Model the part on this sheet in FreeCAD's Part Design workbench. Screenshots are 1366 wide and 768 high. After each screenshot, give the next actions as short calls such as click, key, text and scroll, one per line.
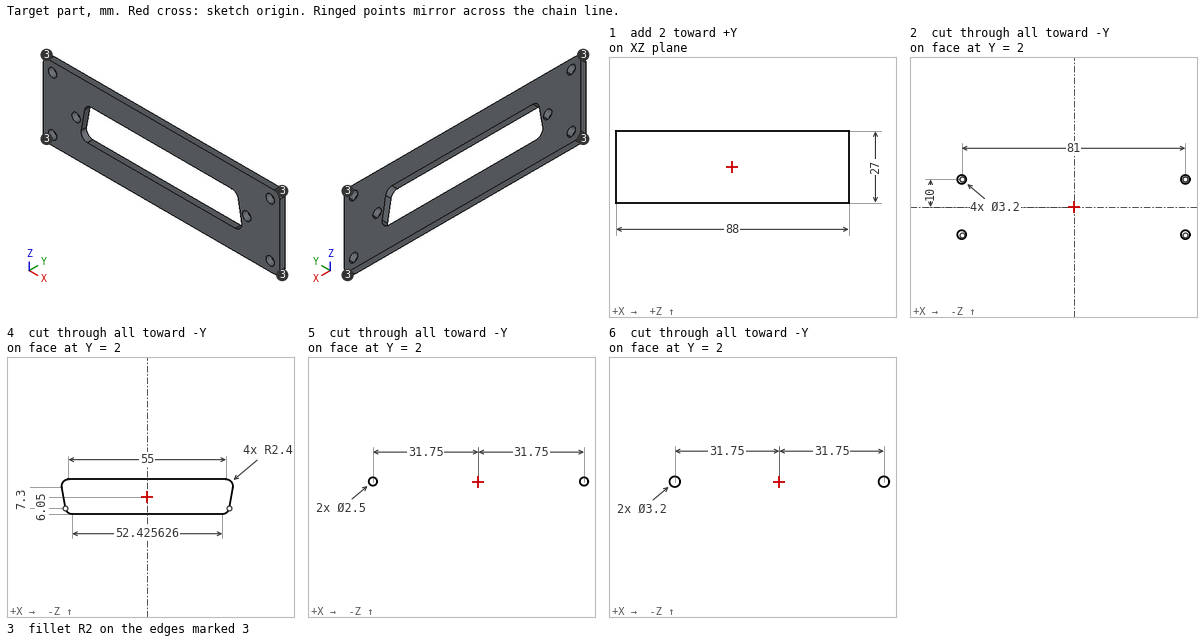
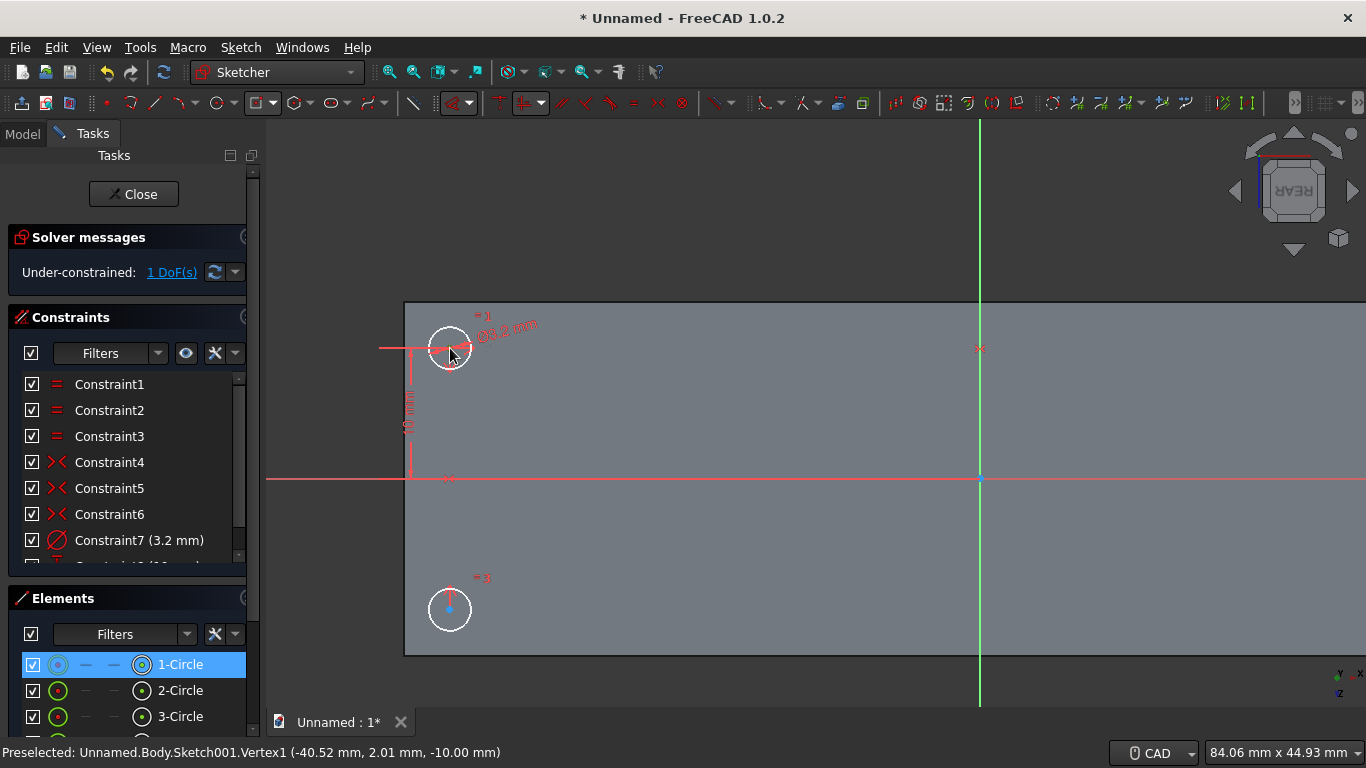
scroll(464, 333, down, 3)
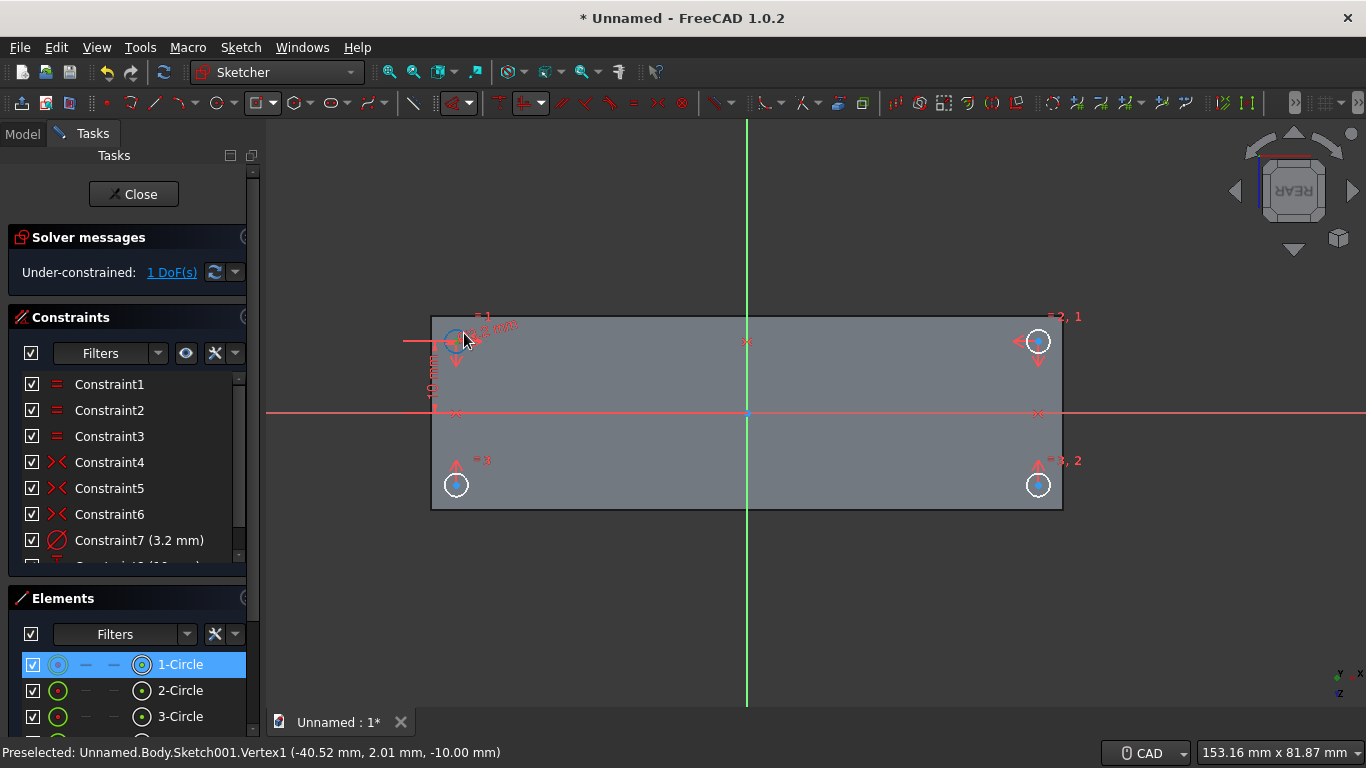
click(1038, 341)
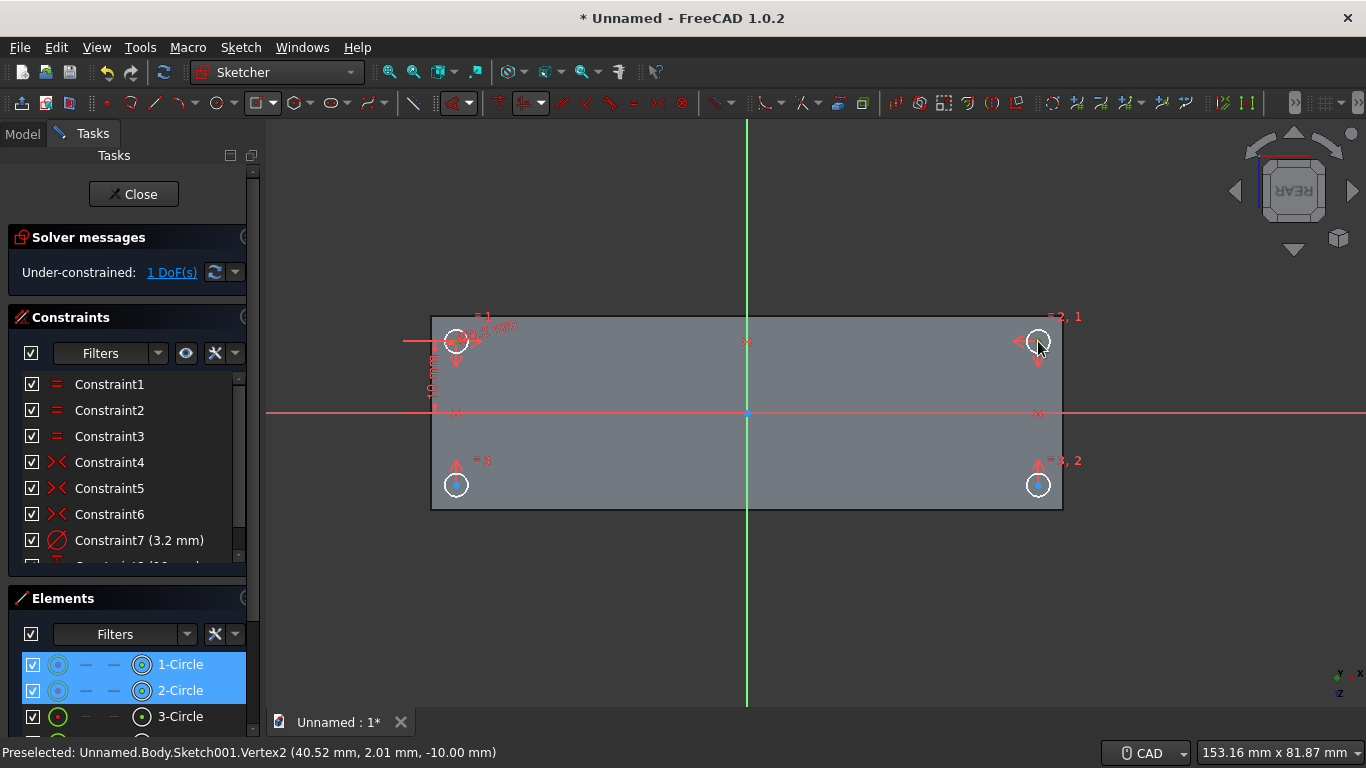
click(472, 104)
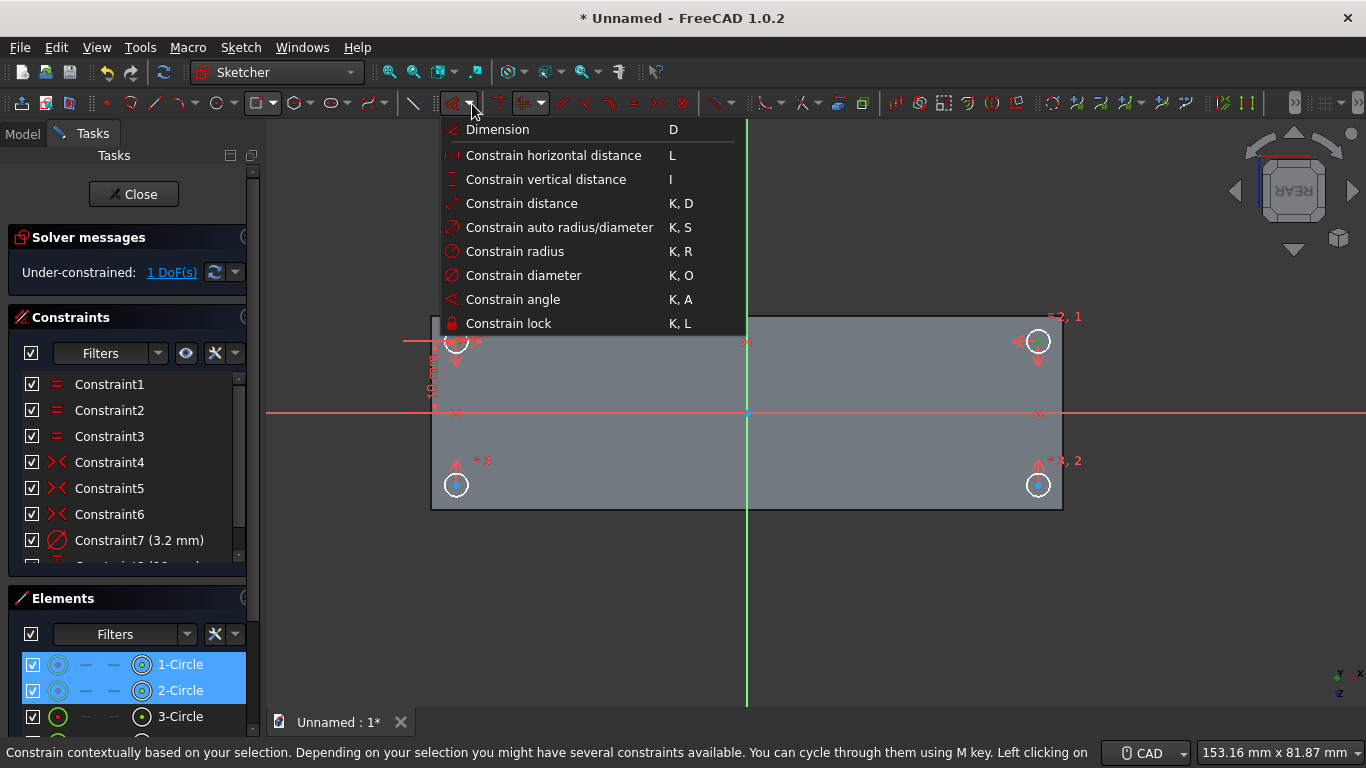
click(593, 155)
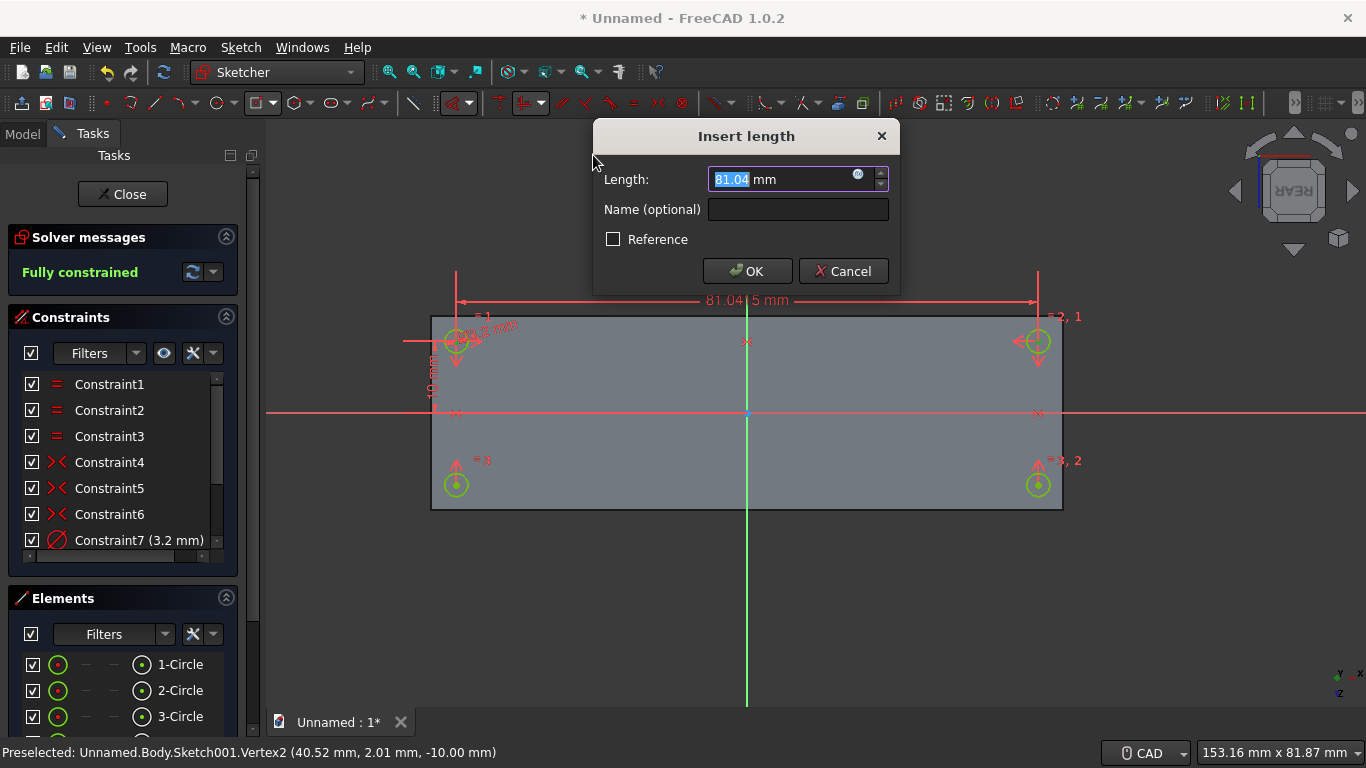
text(81)
key(Return)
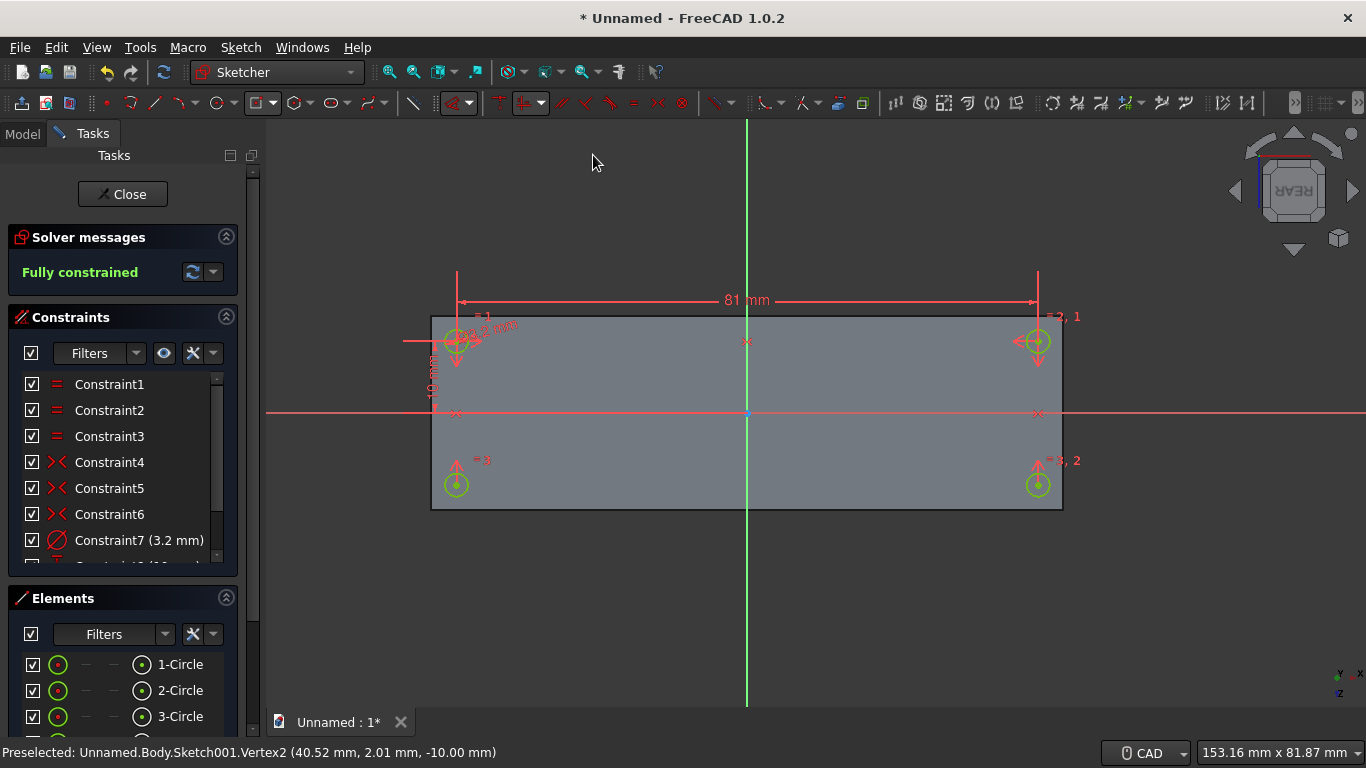
click(123, 194)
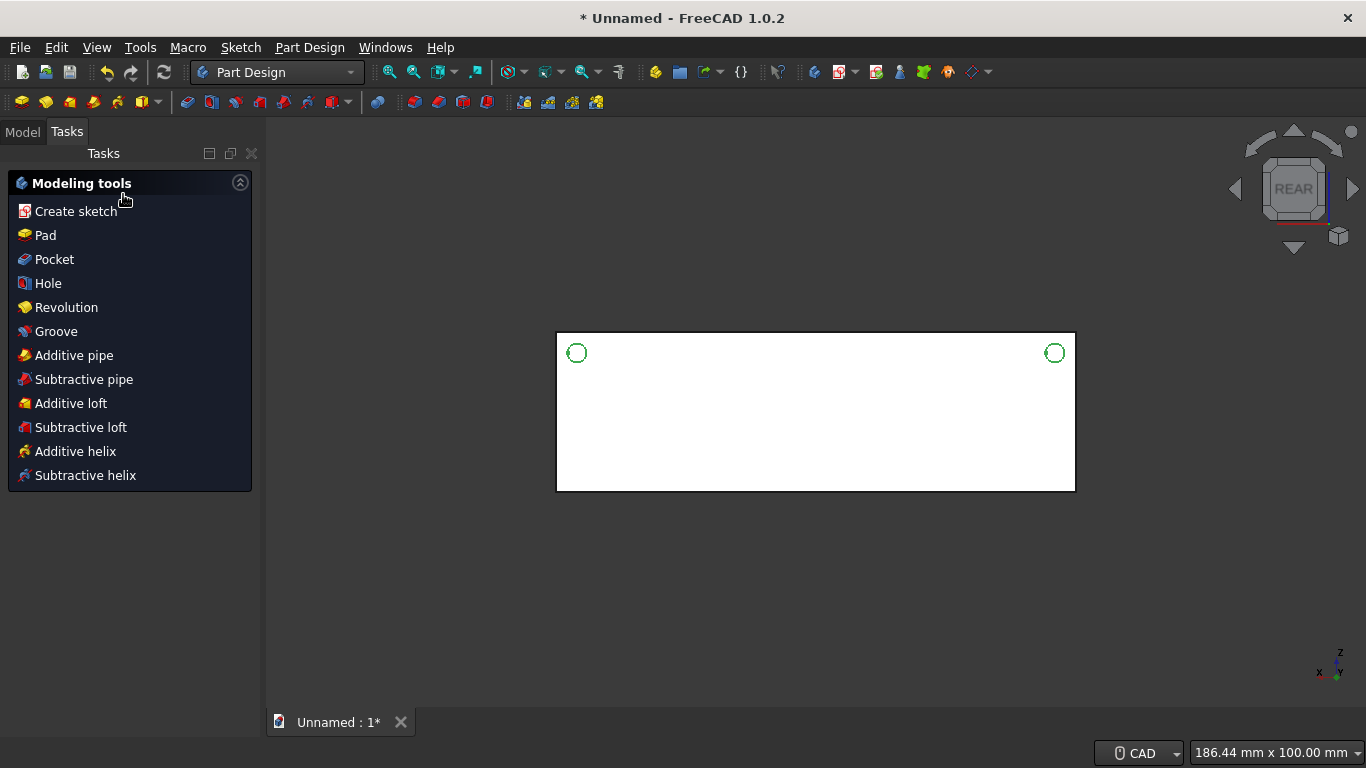
click(188, 102)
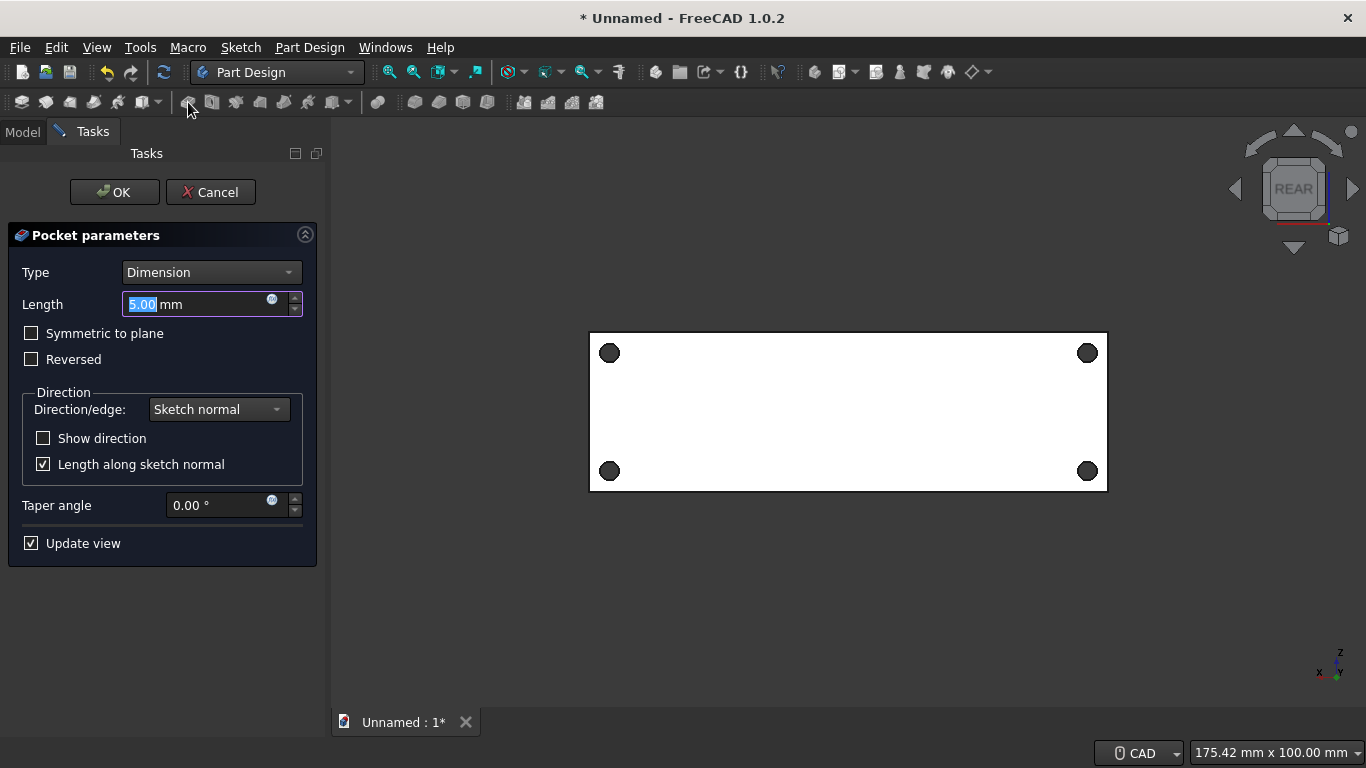
click(212, 272)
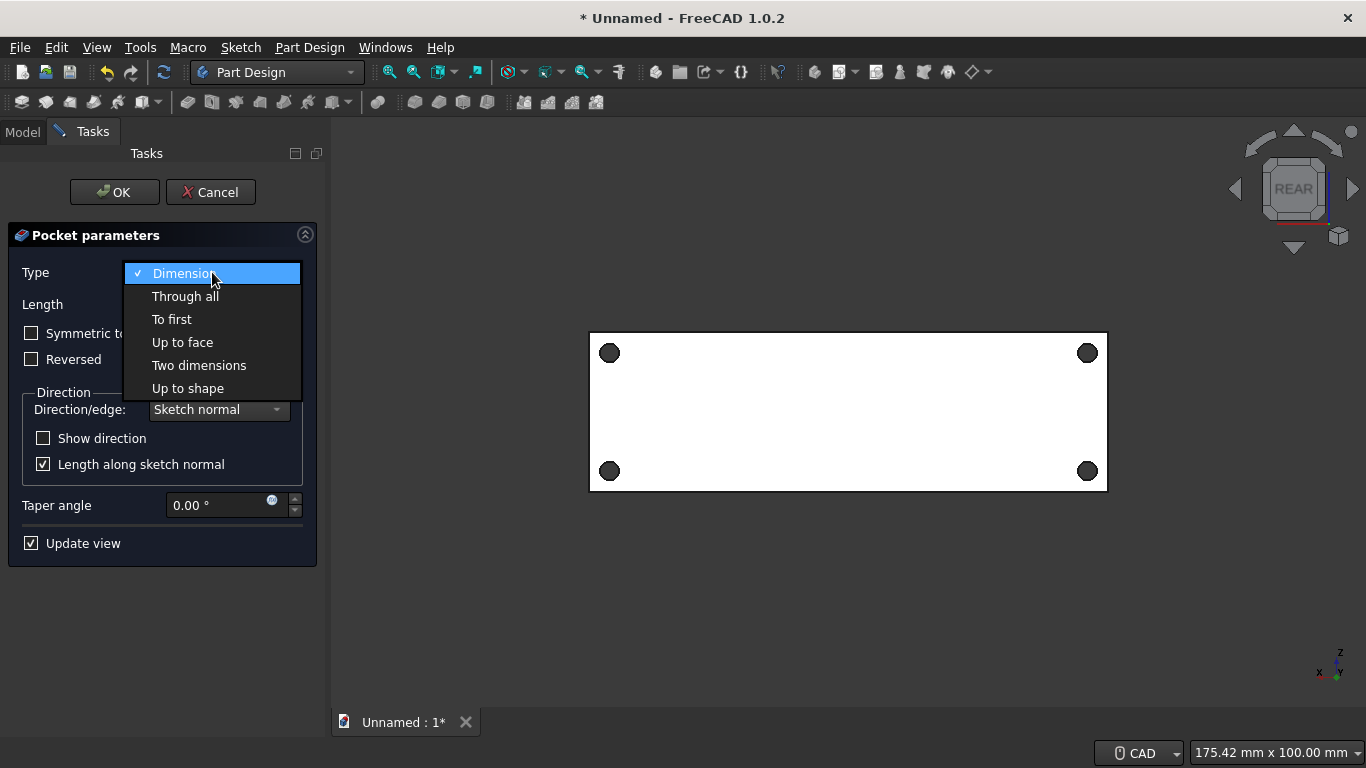
click(212, 296)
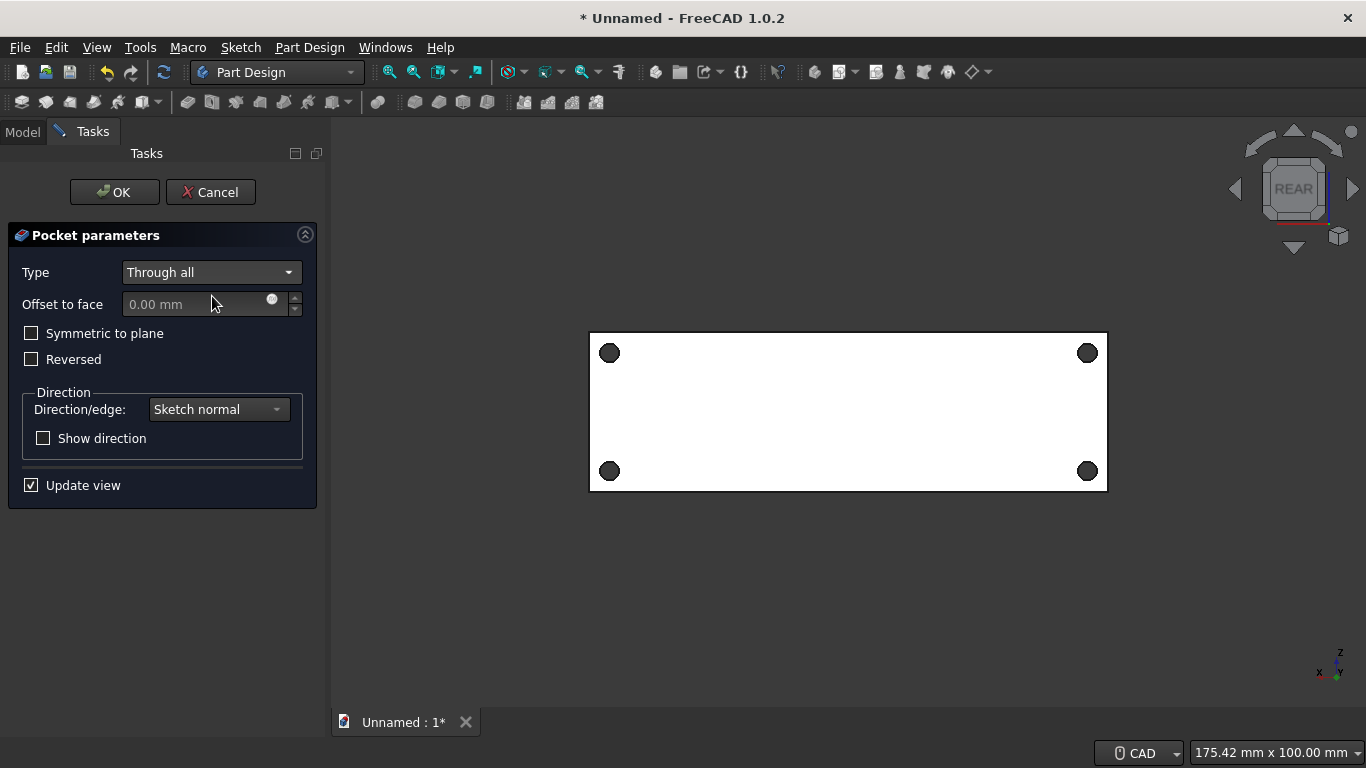
click(115, 192)